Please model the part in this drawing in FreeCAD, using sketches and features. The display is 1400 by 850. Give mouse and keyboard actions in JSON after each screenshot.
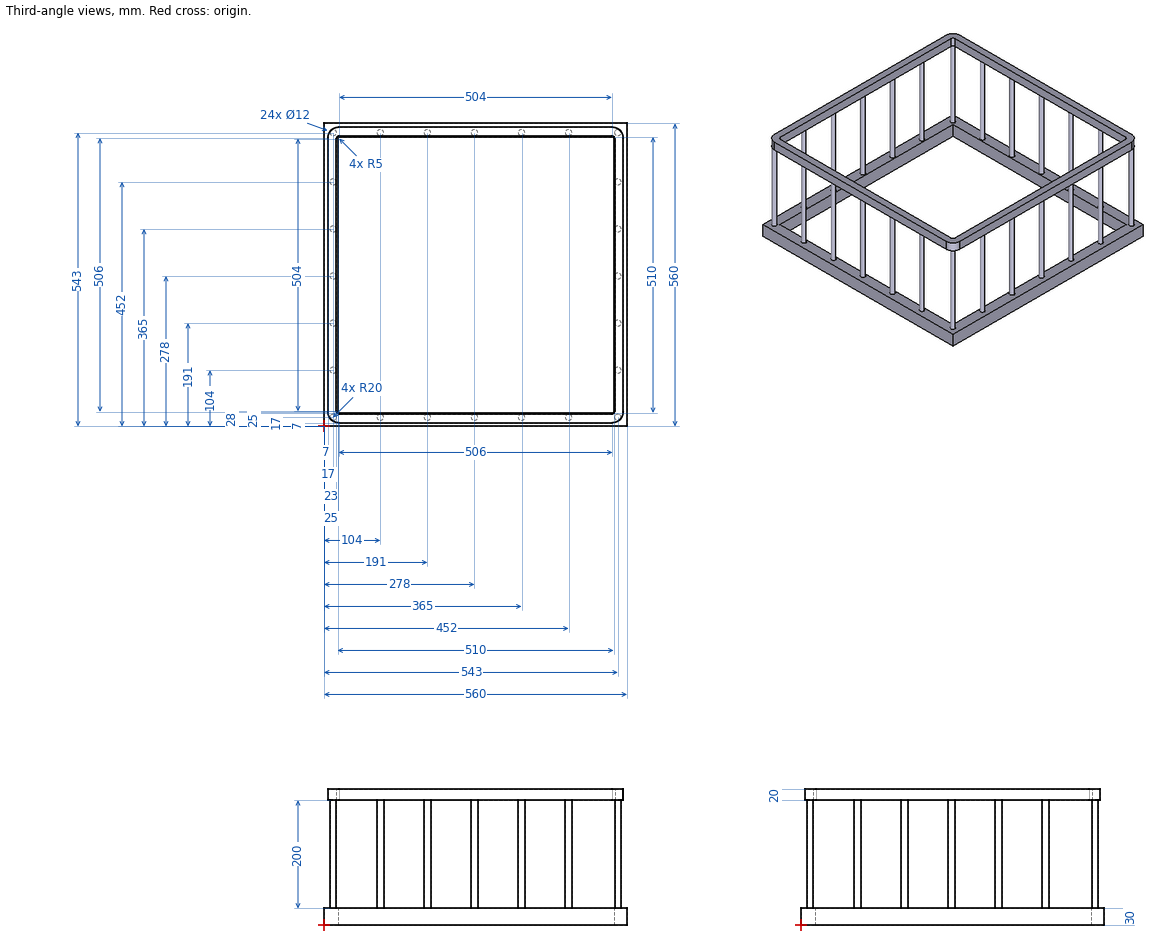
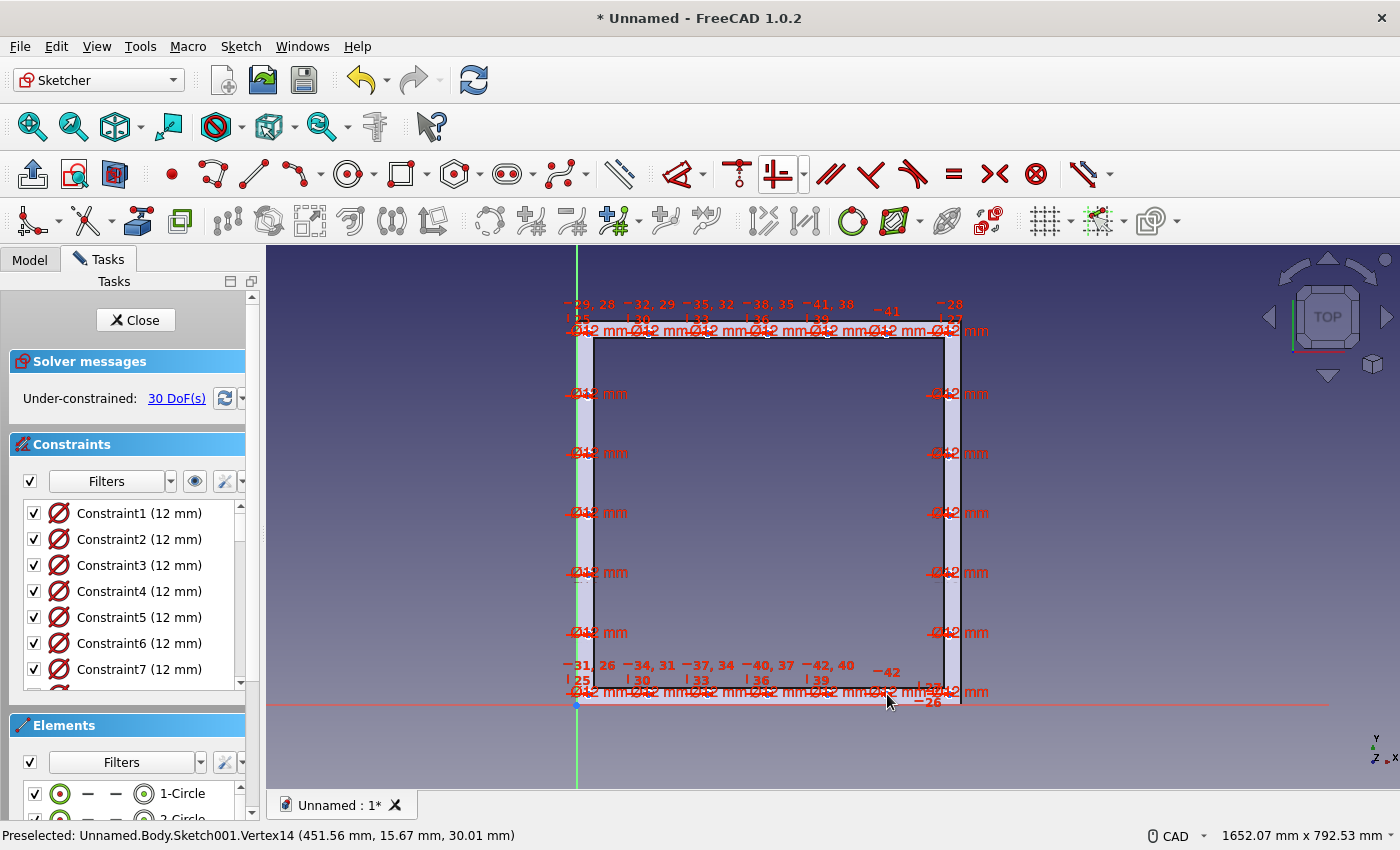
{"action": "left_click", "coordinate": [588, 694]}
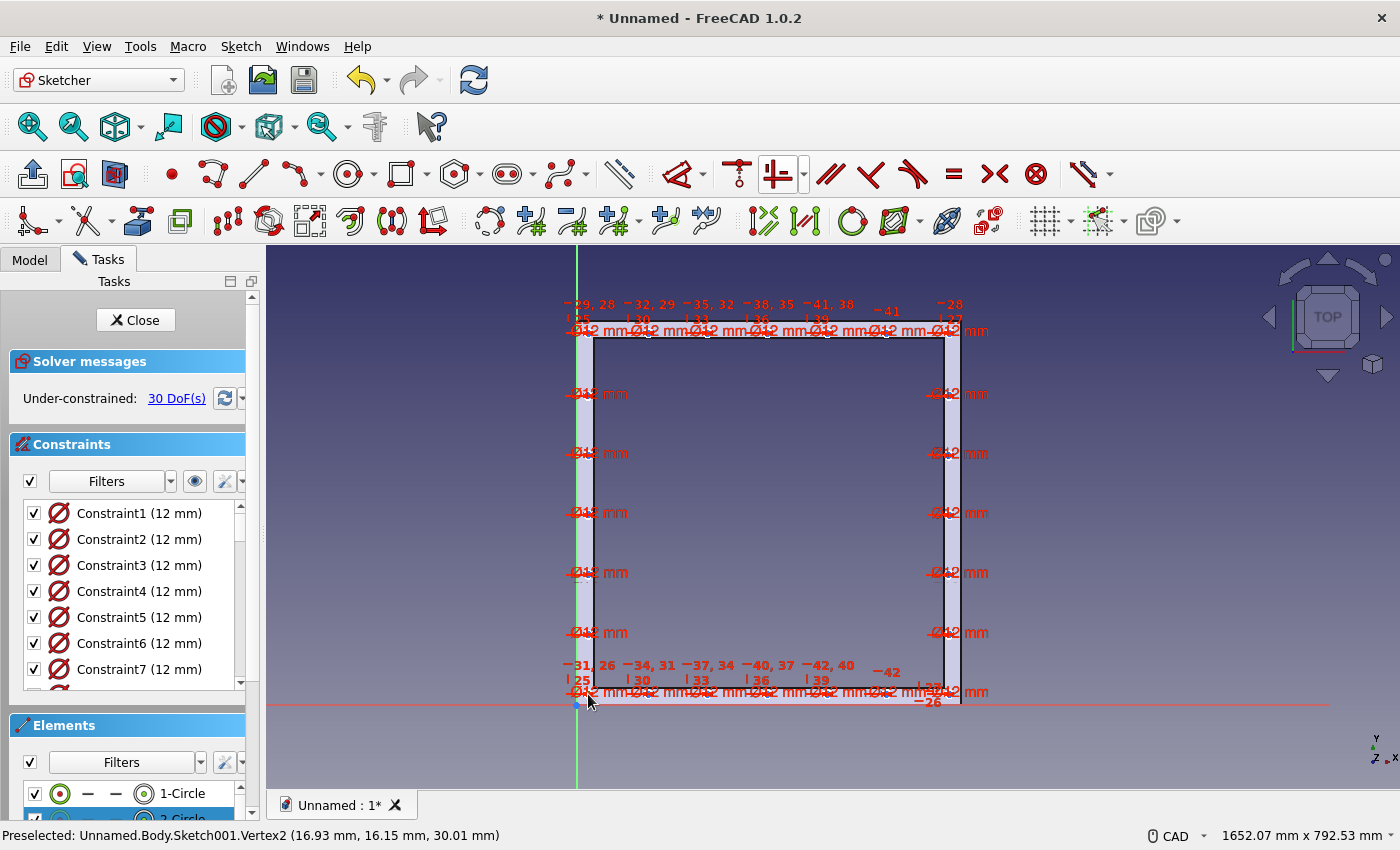
{"action": "left_click", "coordinate": [588, 635]}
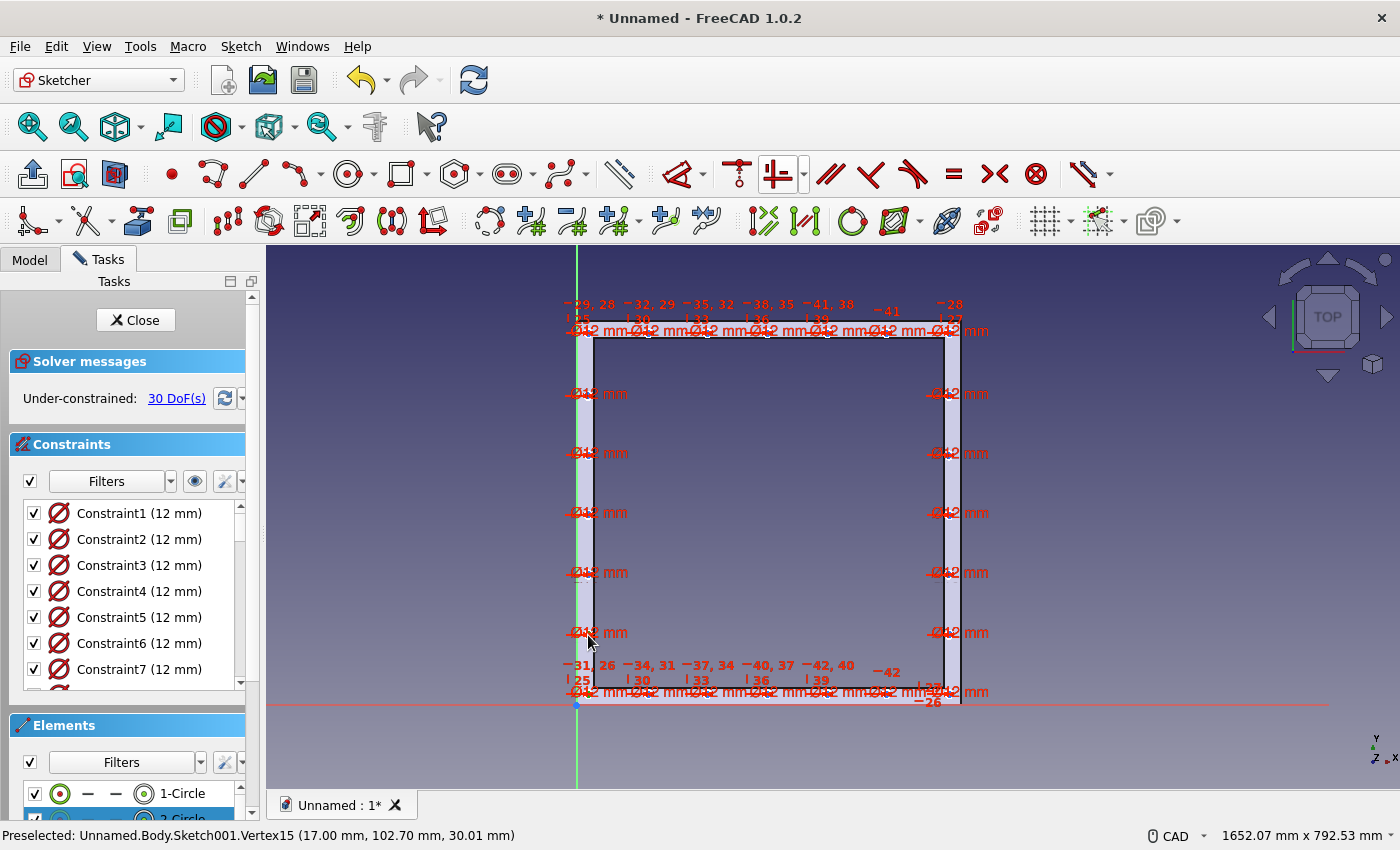
{"action": "key", "text": "v"}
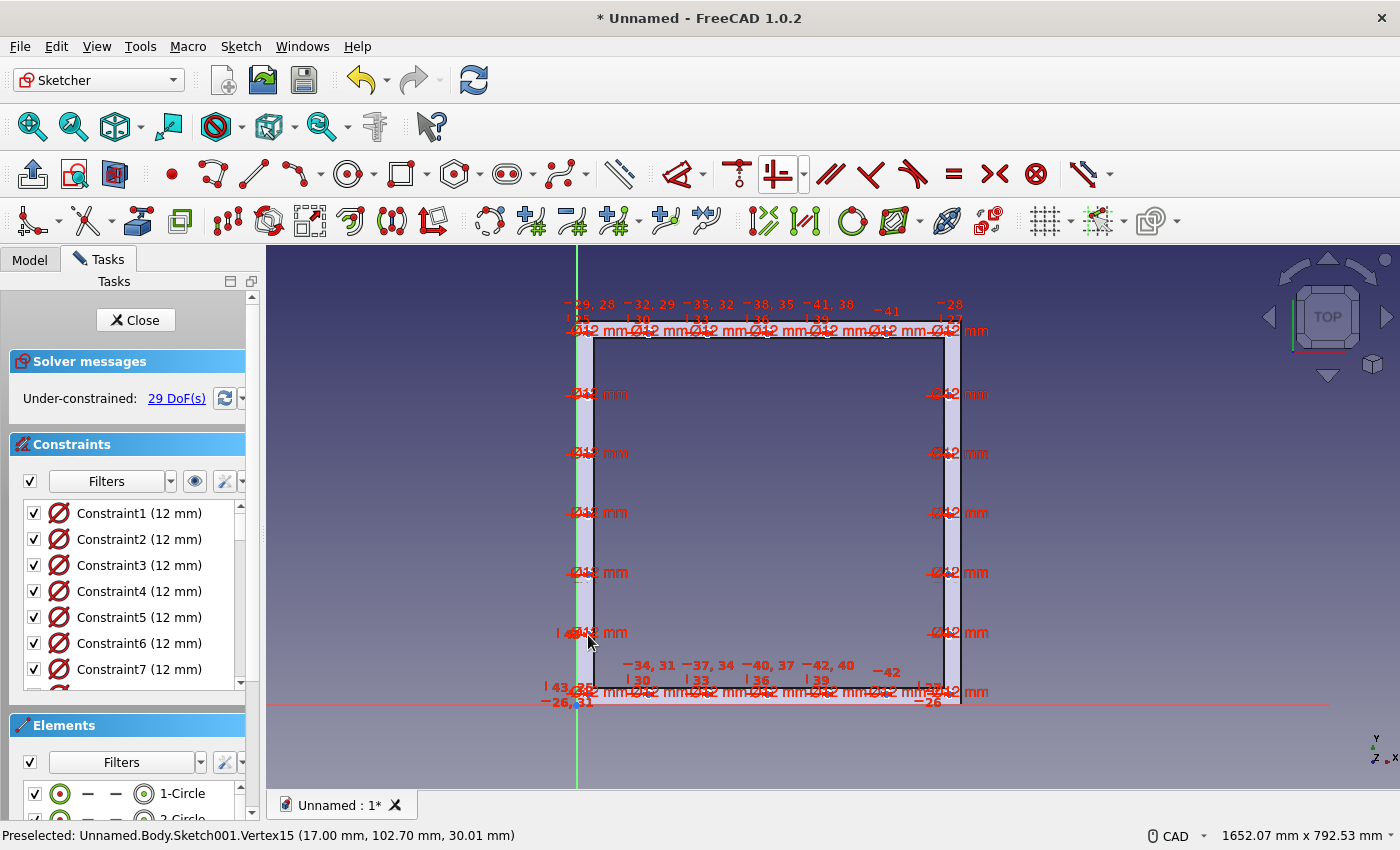
{"action": "left_click", "coordinate": [949, 694]}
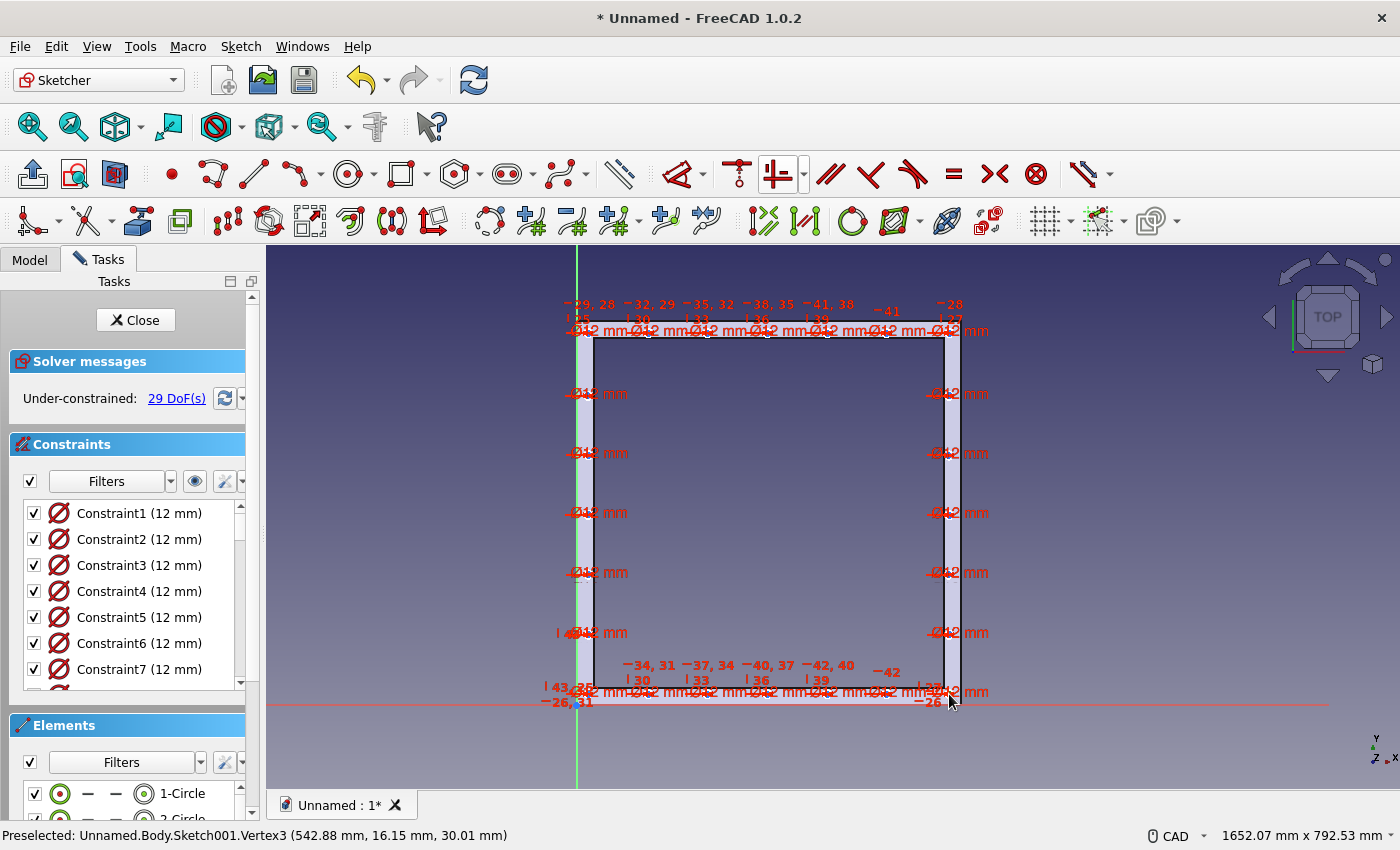
{"action": "left_click", "coordinate": [949, 635]}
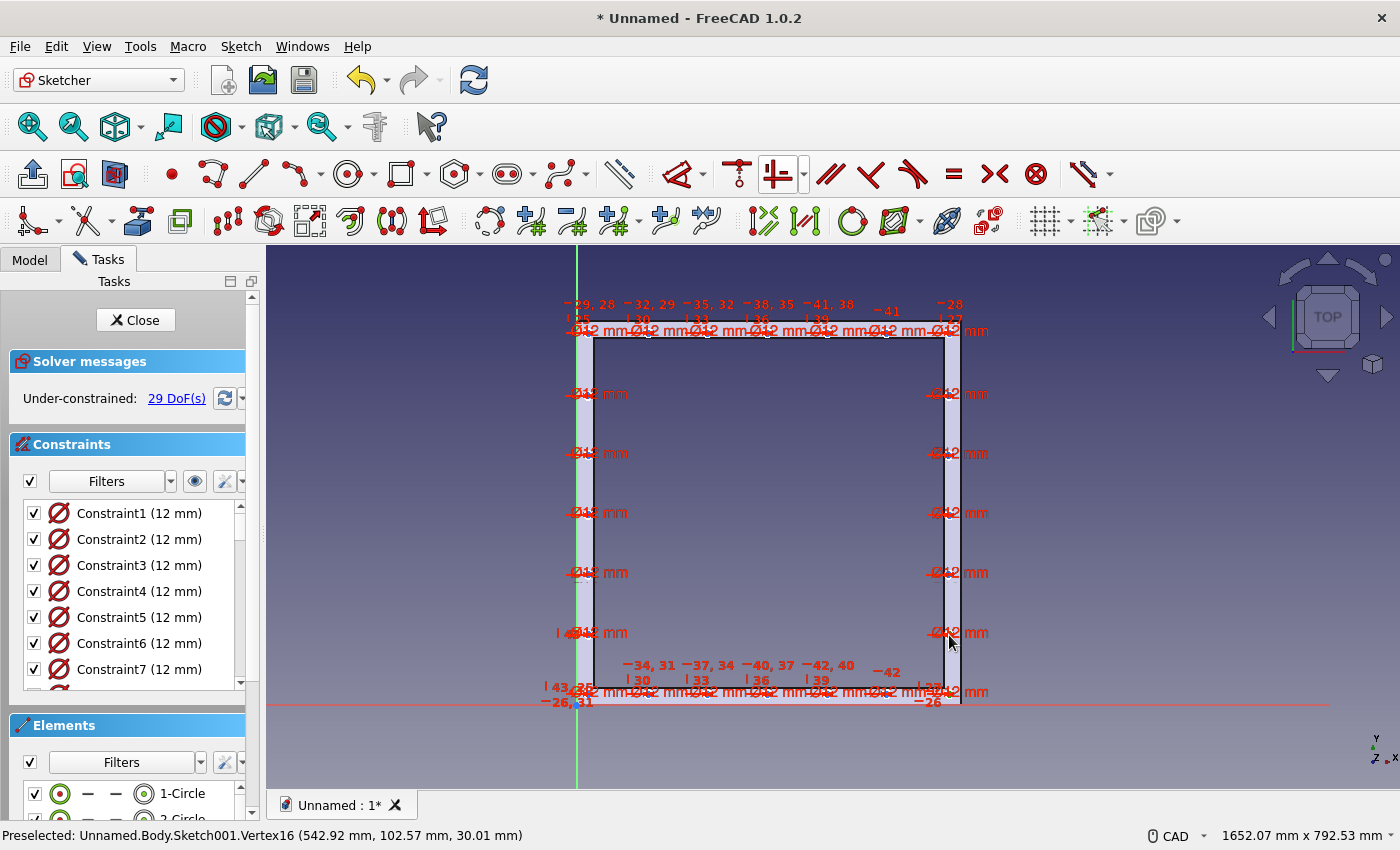
{"action": "left_click", "coordinate": [804, 174]}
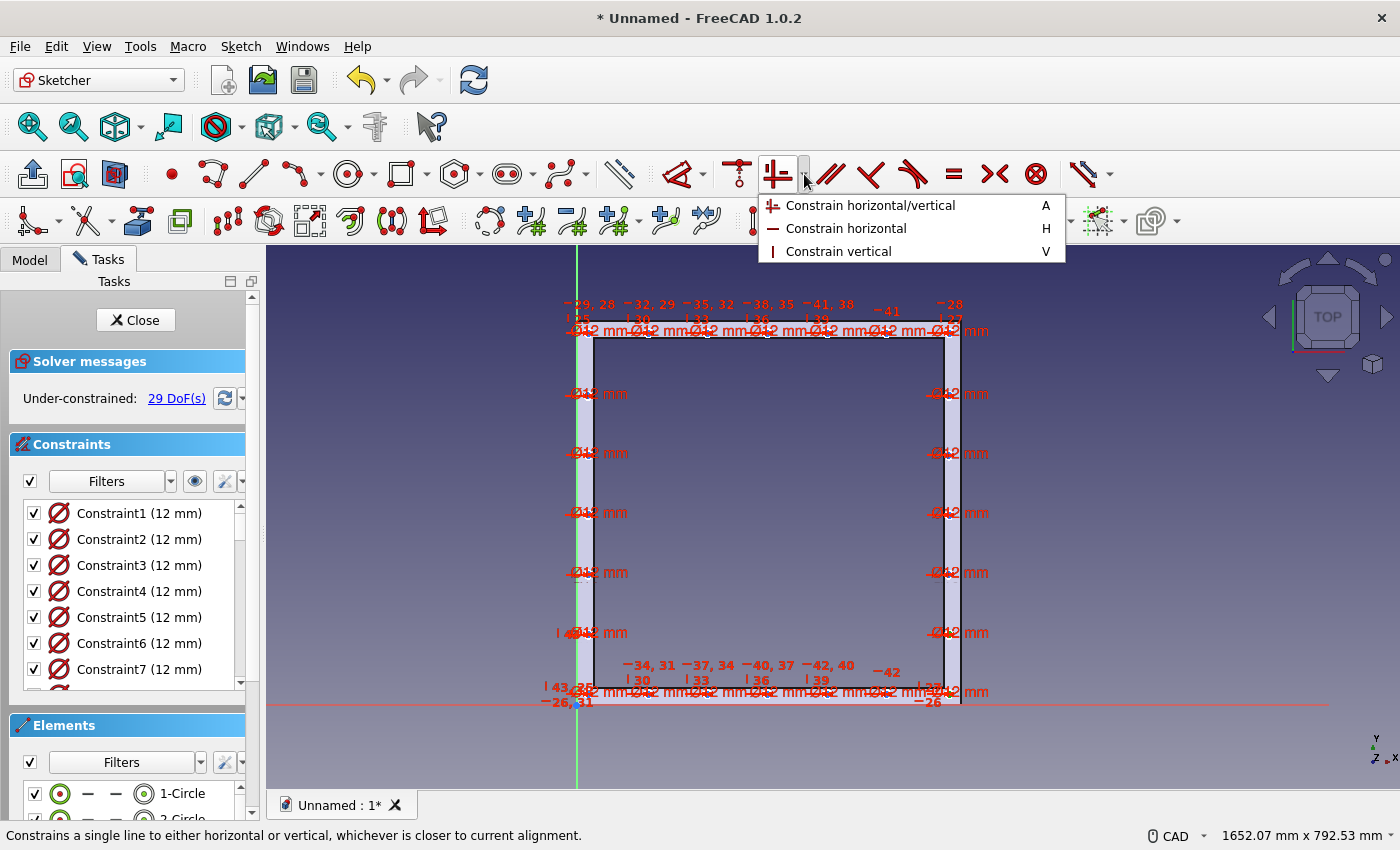
{"action": "left_click", "coordinate": [912, 252]}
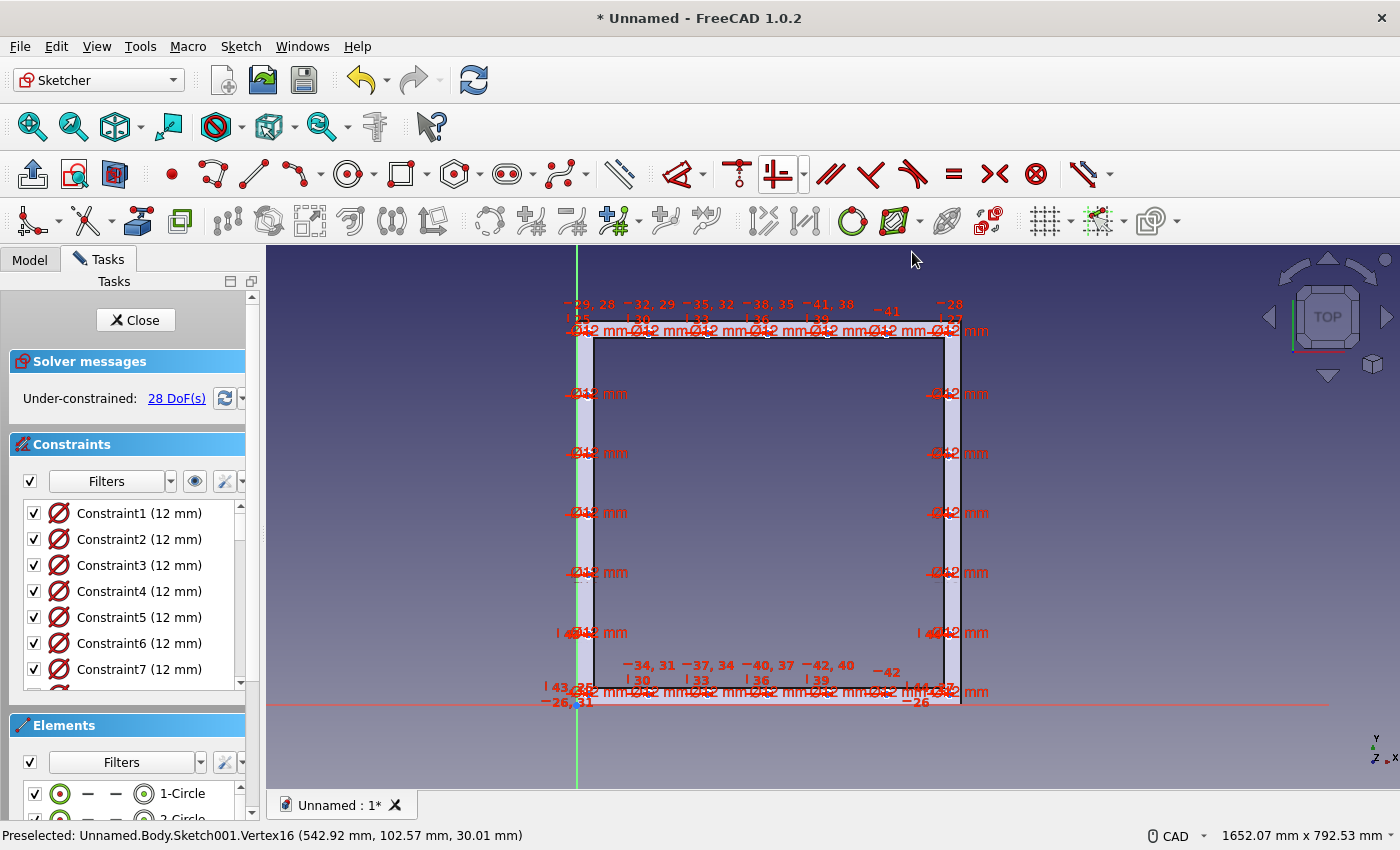
{"action": "left_click", "coordinate": [588, 635]}